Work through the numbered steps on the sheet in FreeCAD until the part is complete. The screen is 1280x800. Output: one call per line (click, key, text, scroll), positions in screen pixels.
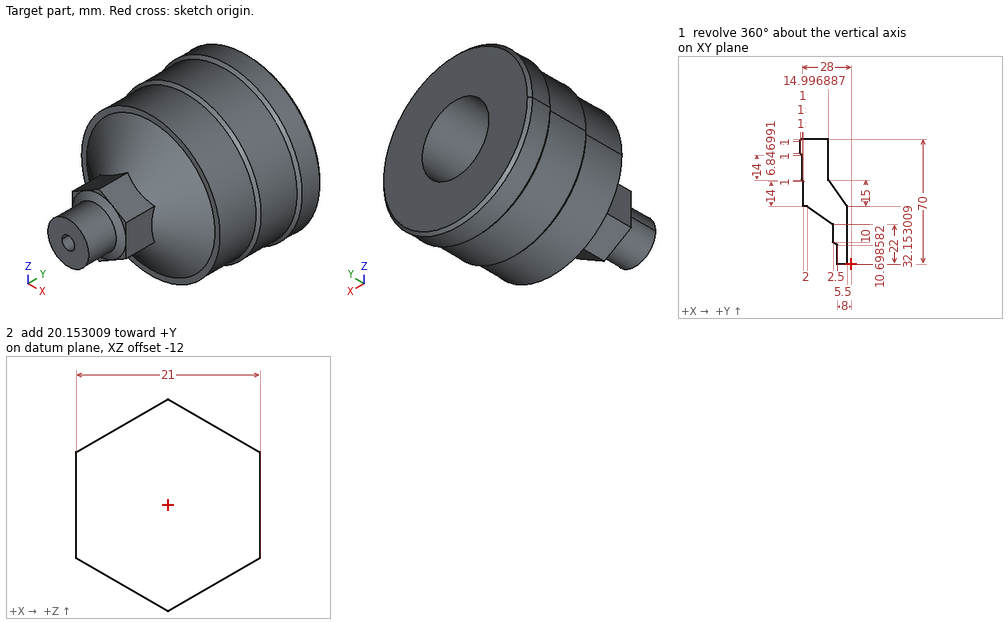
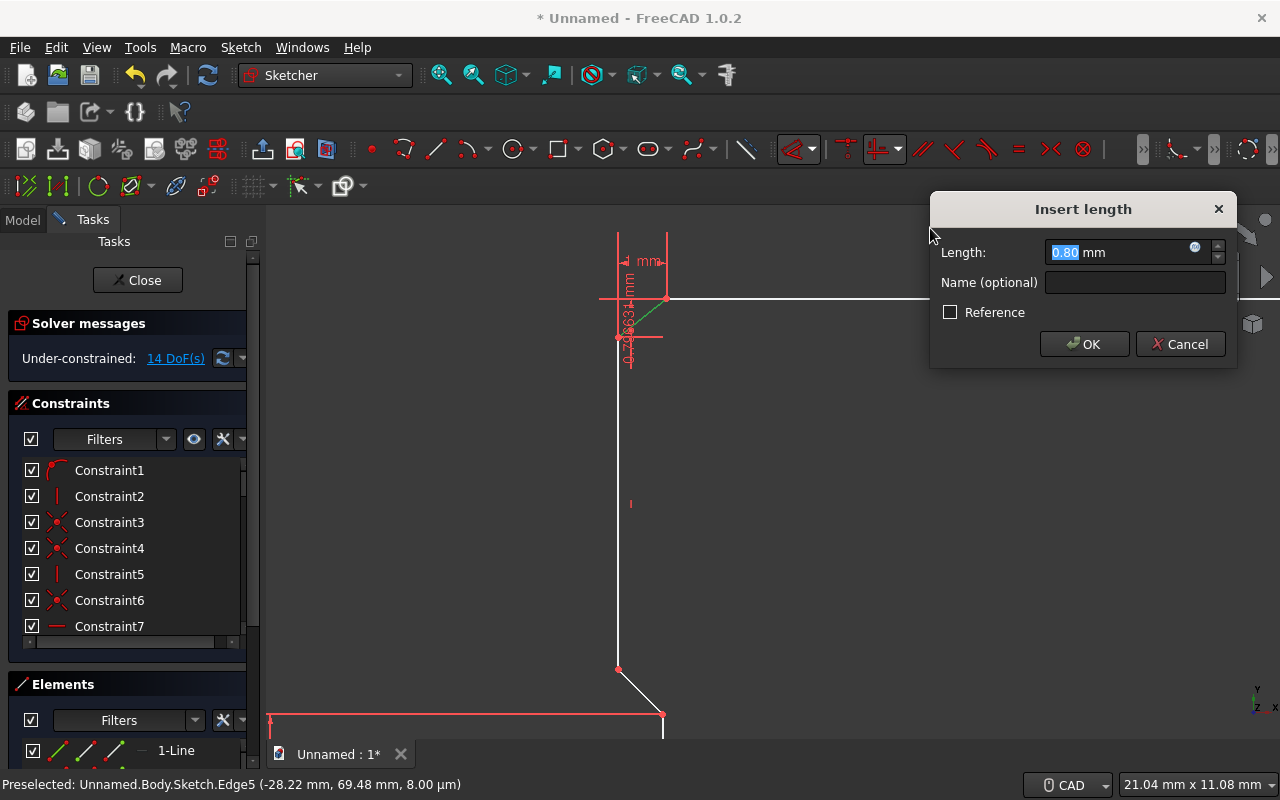
text(1)
key(Return)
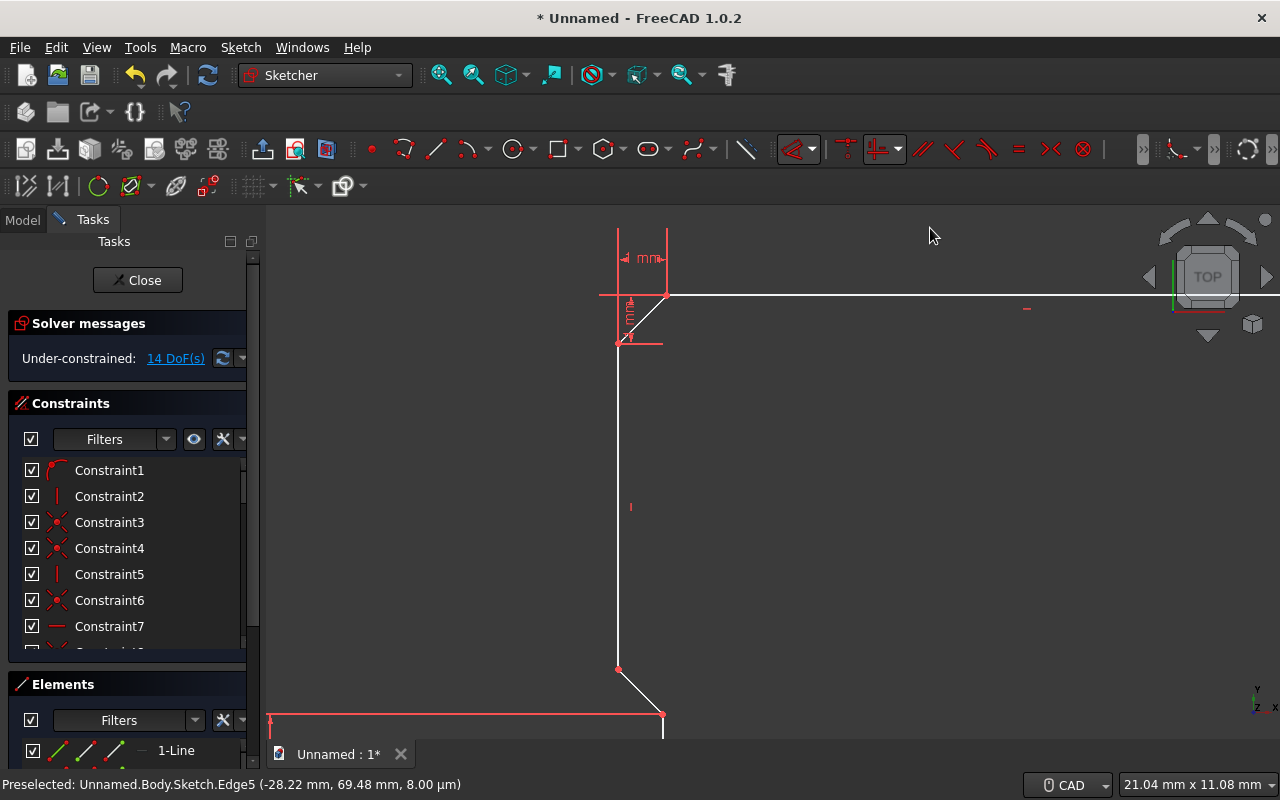
click(632, 683)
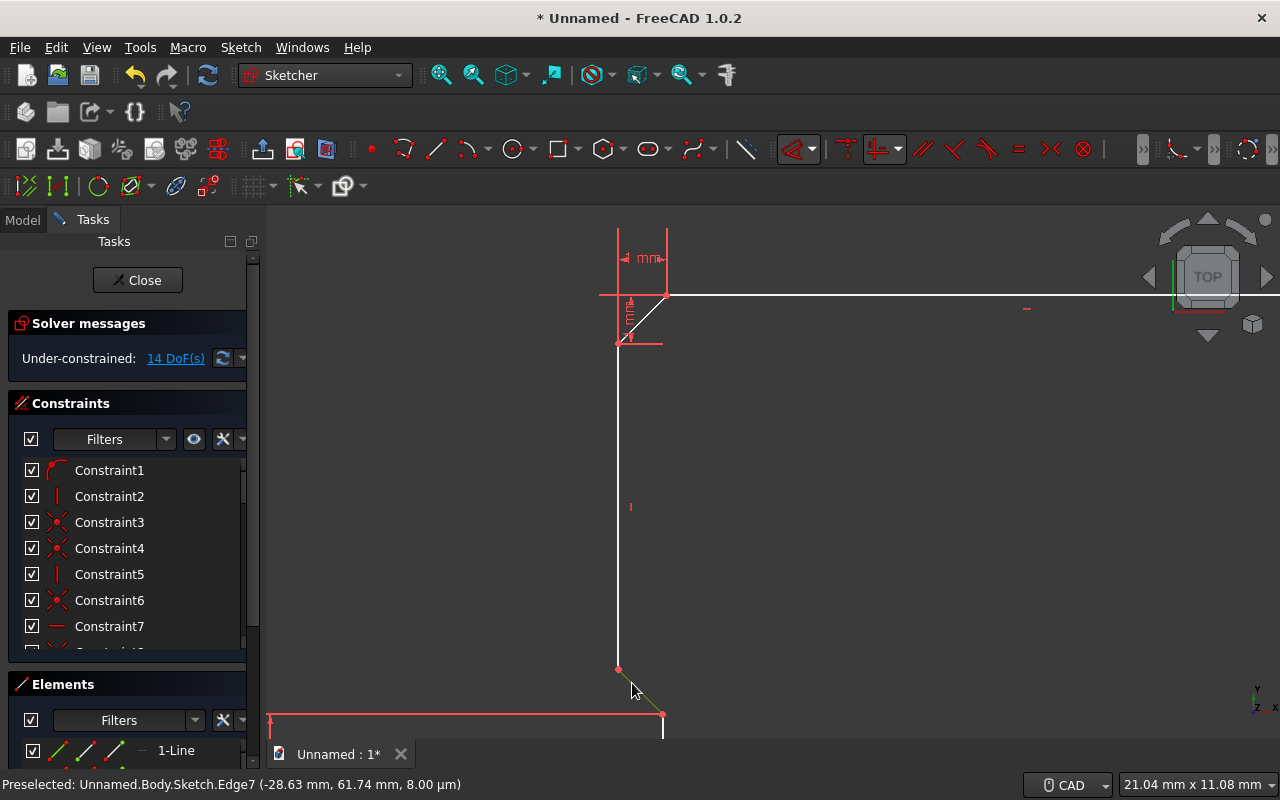
key(l)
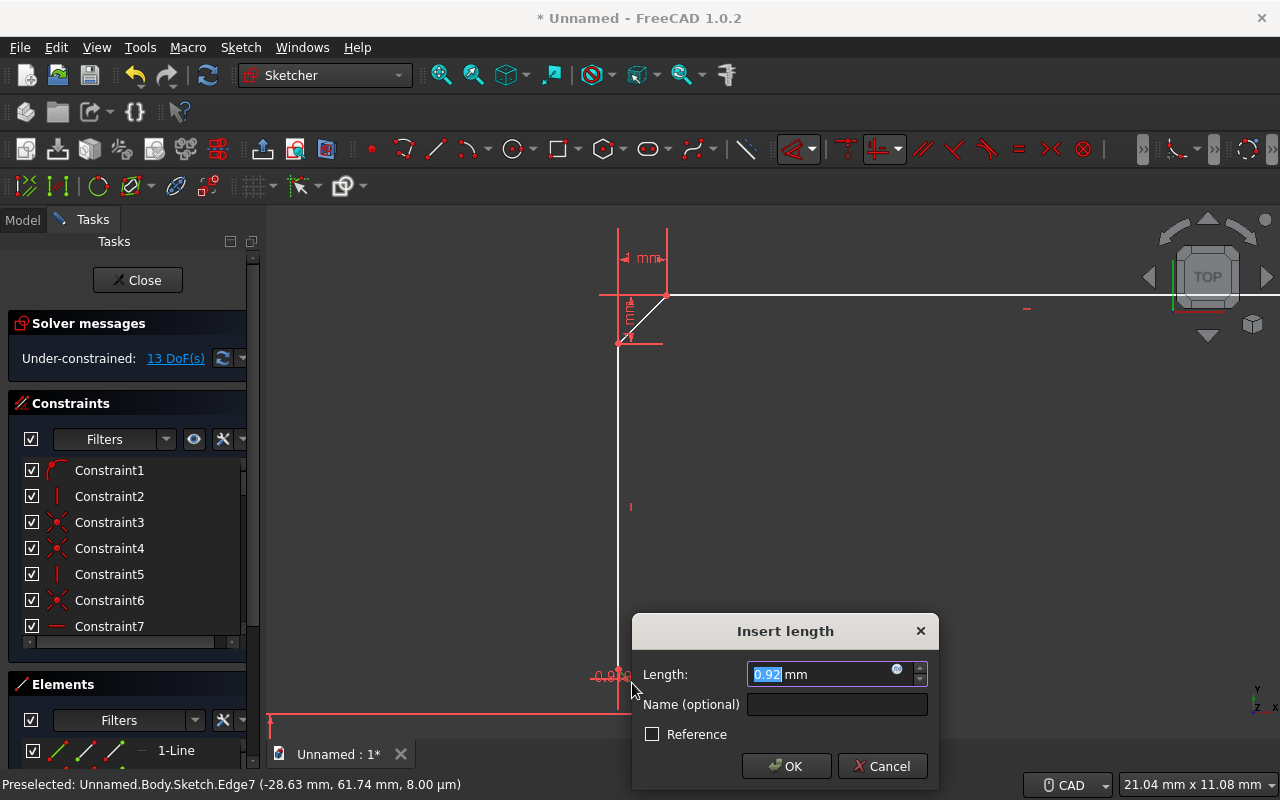
text(1)
key(Return)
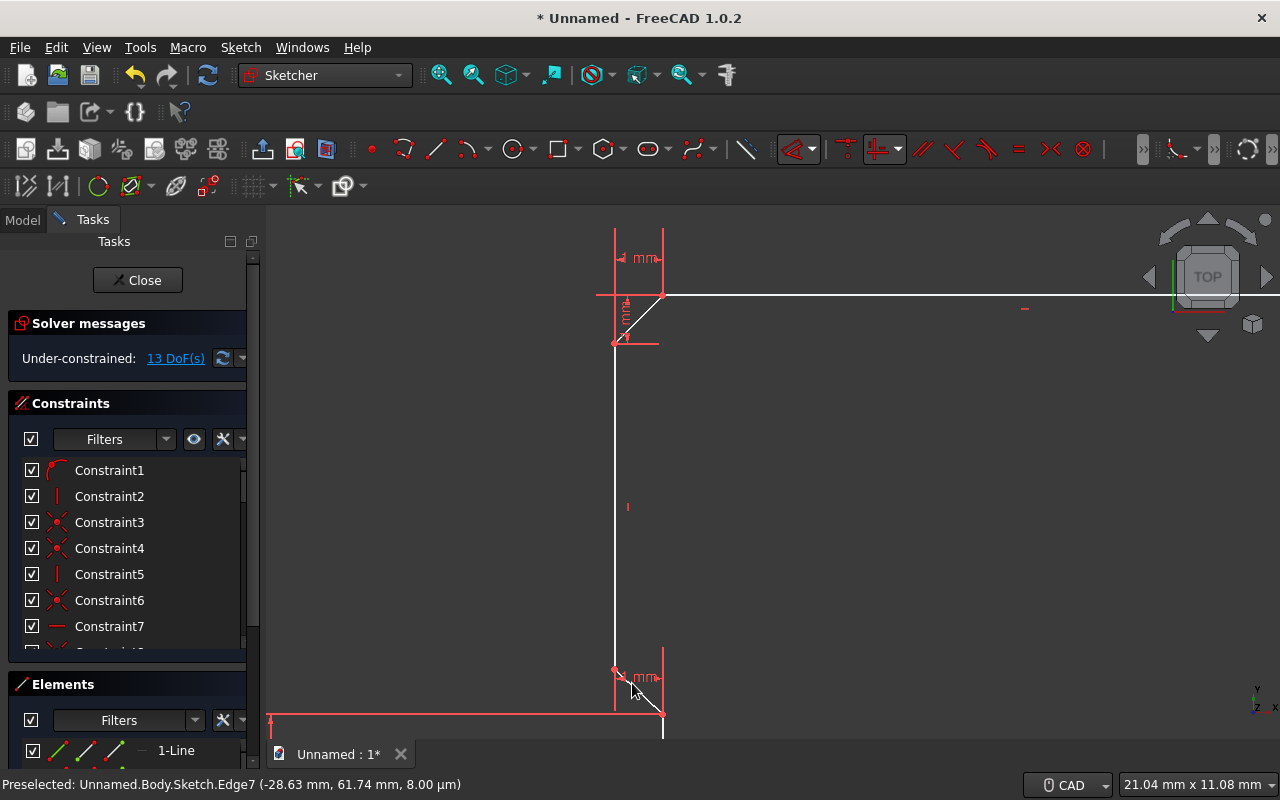
click(649, 701)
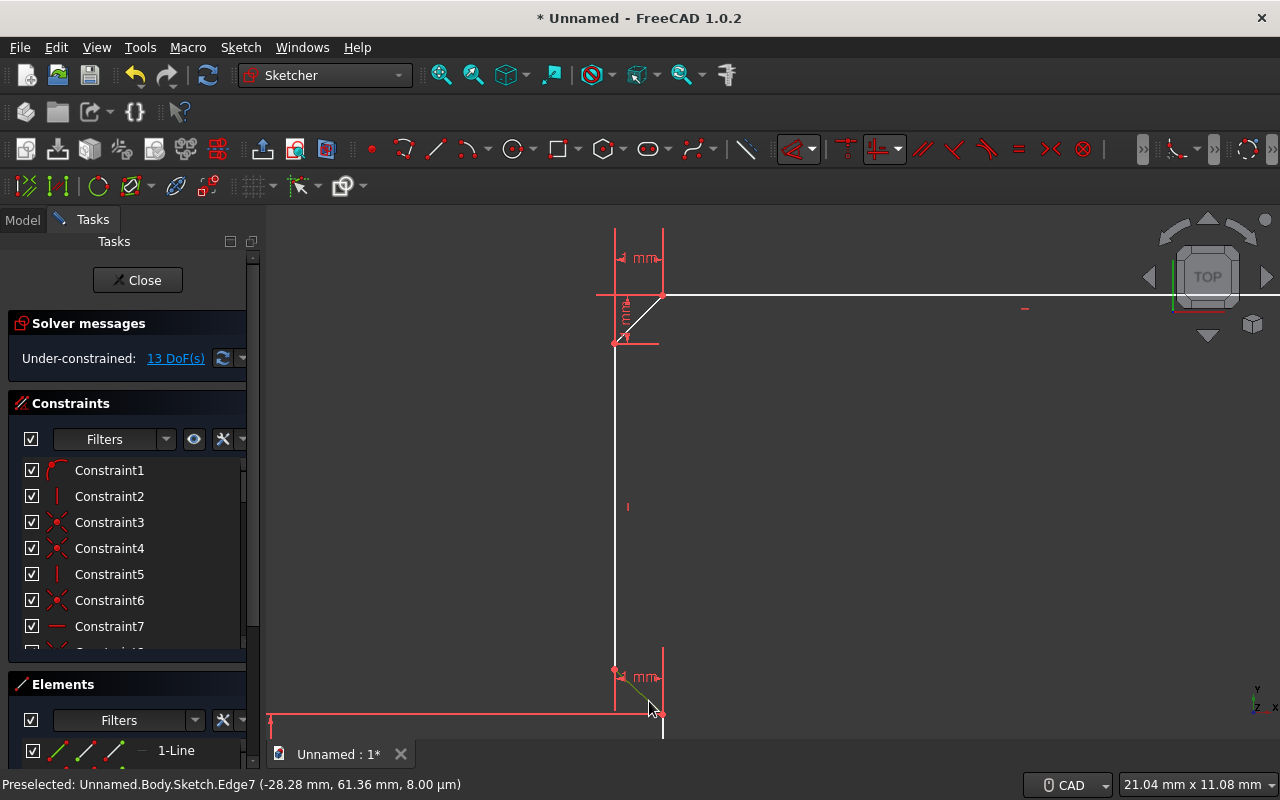
key(i)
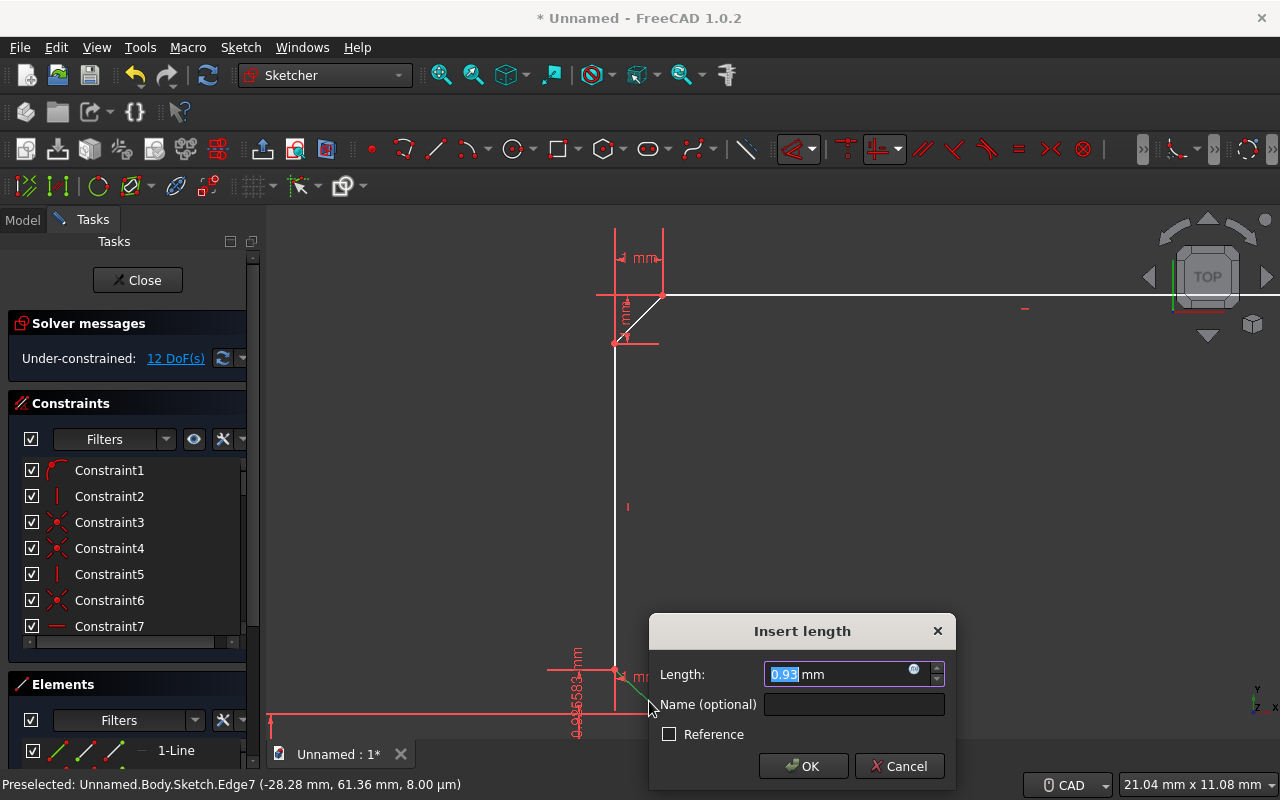
text(1)
key(Return)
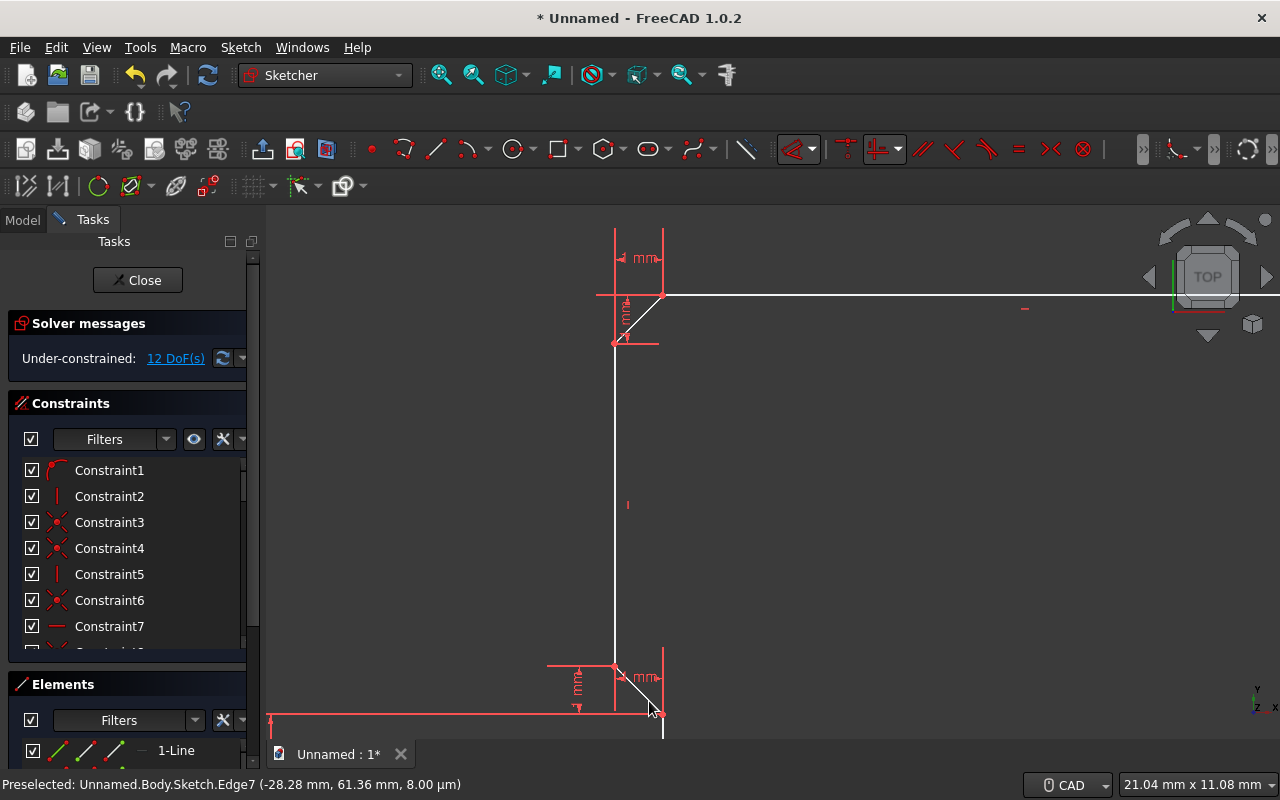
scroll(644, 322, down, 12)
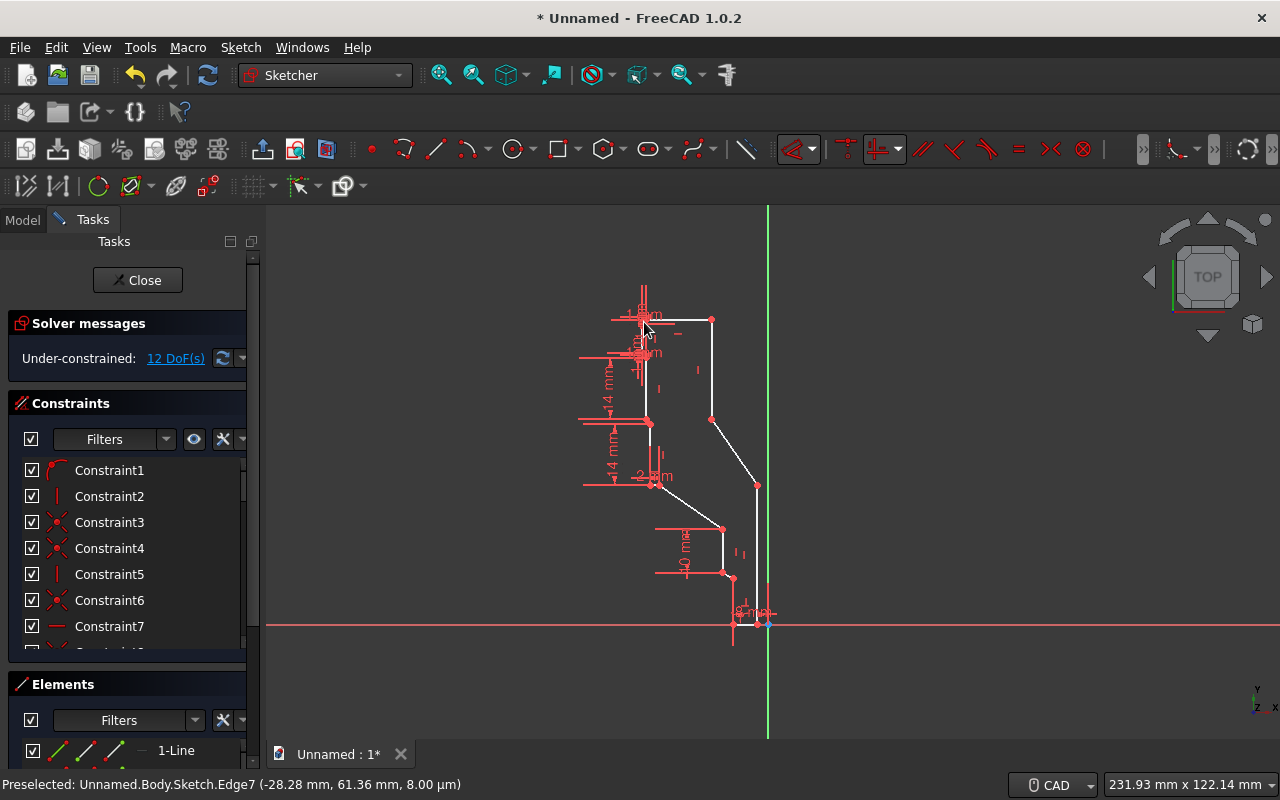
scroll(647, 421, up, 12)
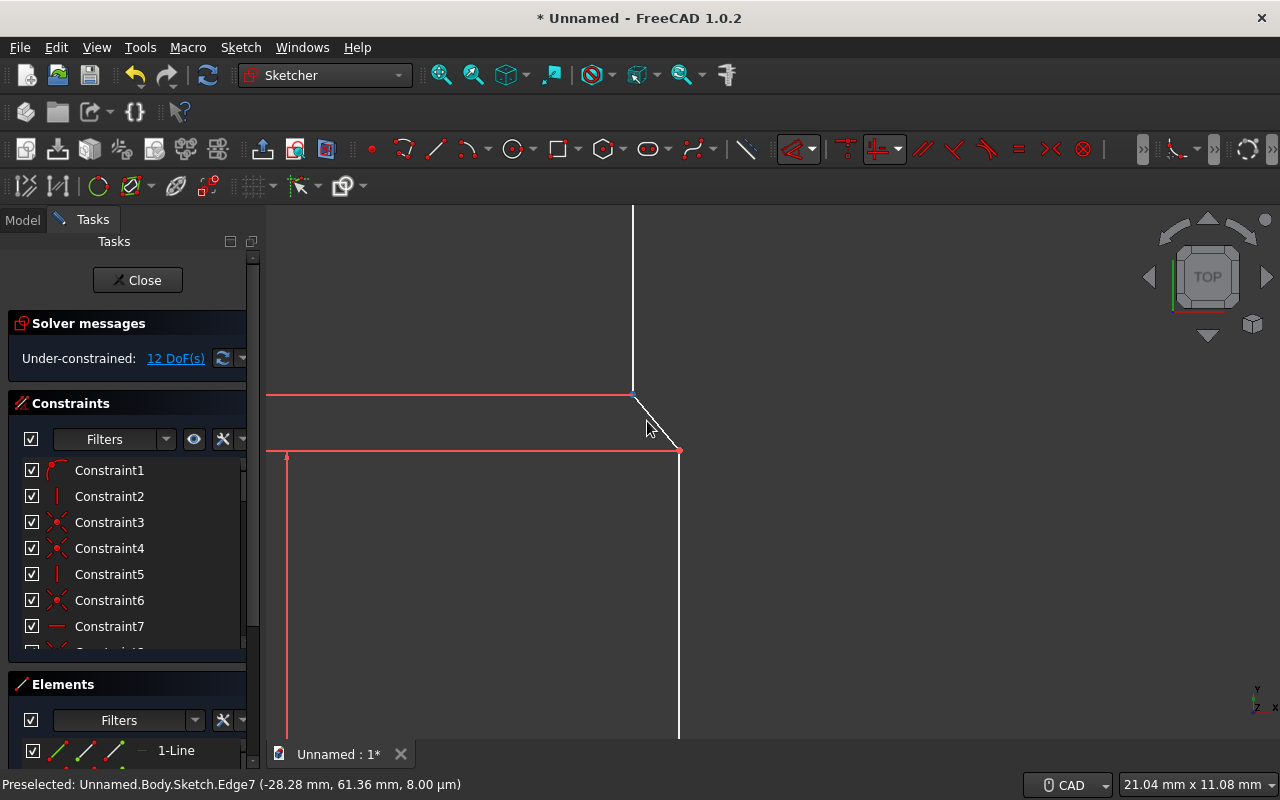
click(647, 412)